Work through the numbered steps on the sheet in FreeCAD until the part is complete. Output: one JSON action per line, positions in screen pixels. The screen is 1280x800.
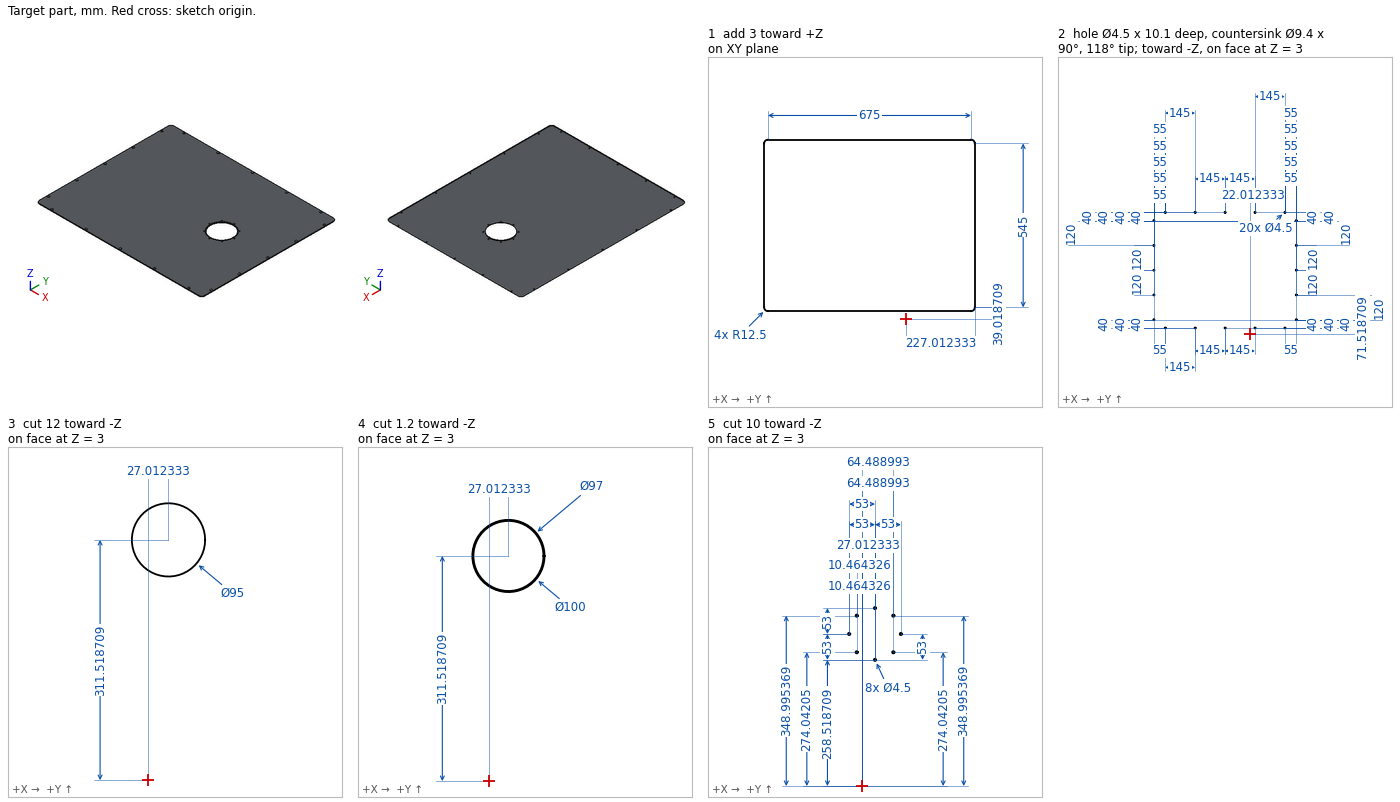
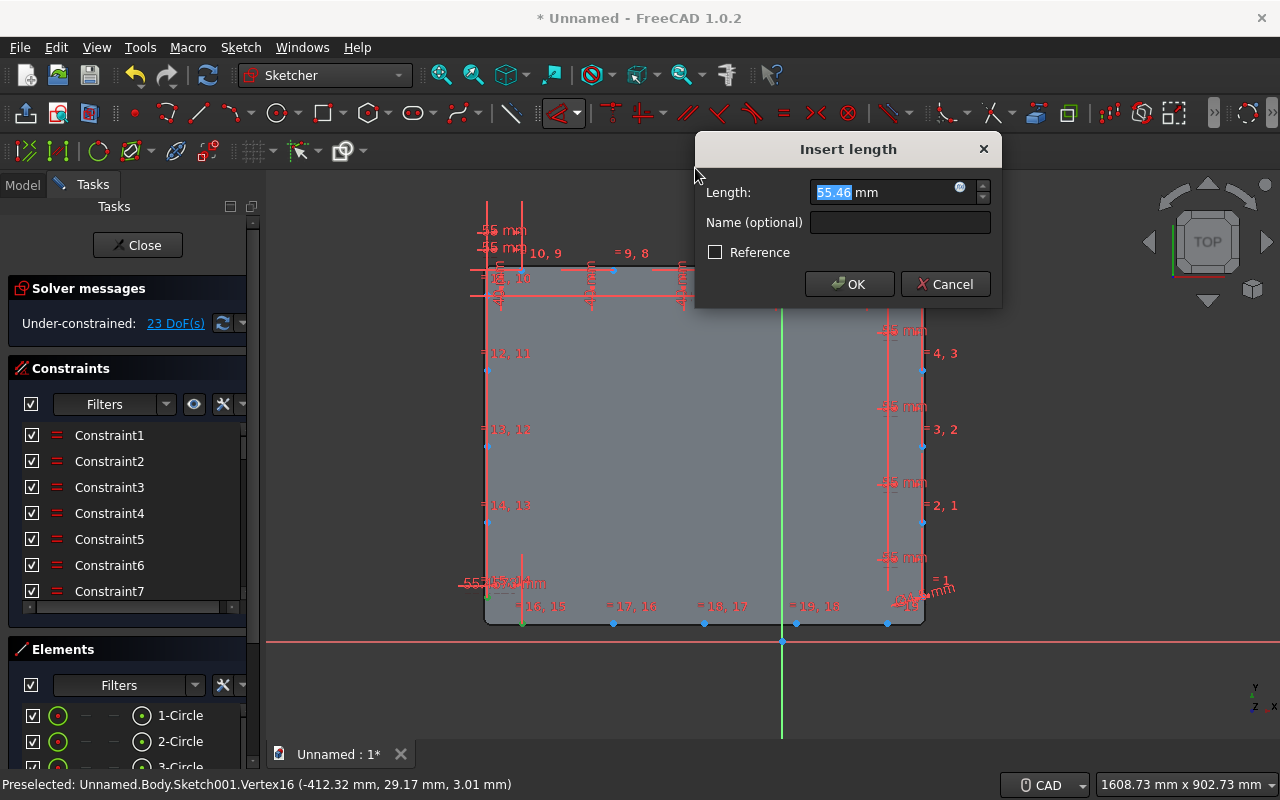
{"action": "type", "text": "55"}
{"action": "key", "text": "Return"}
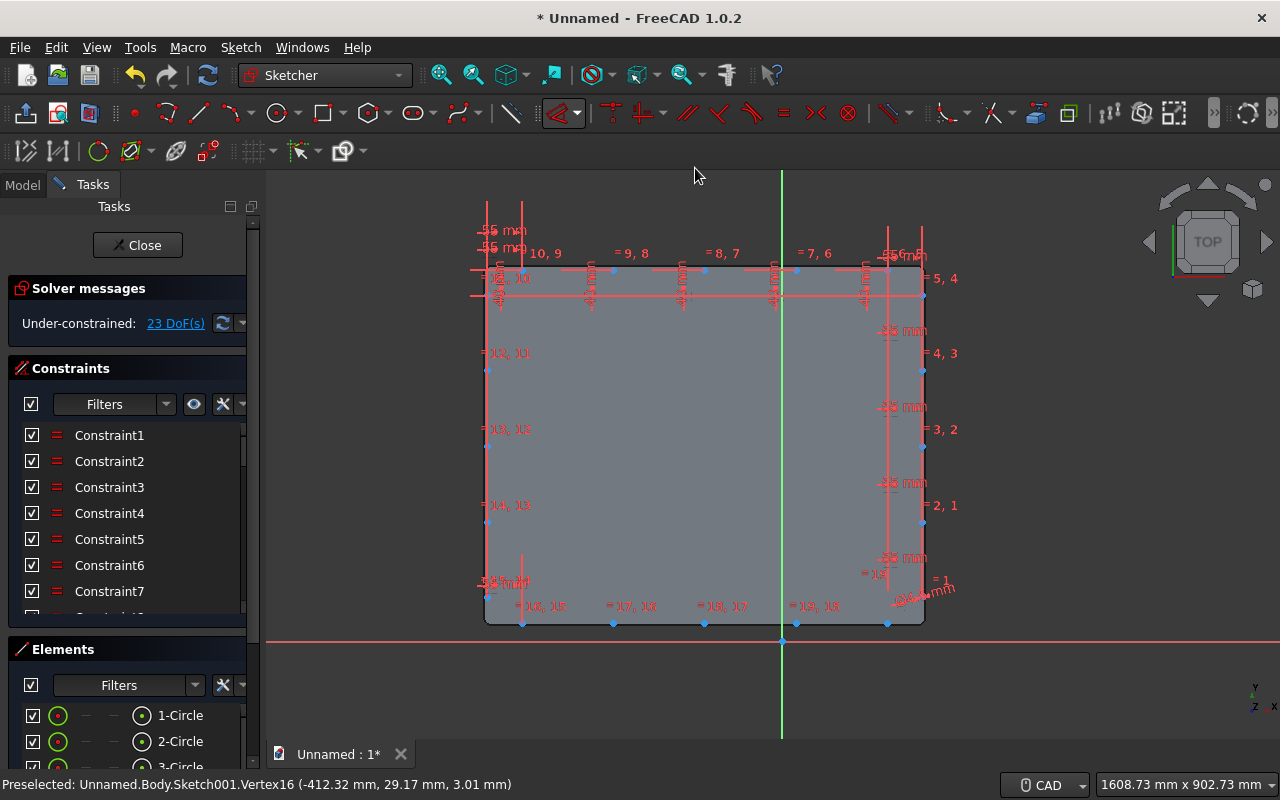
{"action": "scroll", "coordinate": [487, 597], "scroll_direction": "up", "scroll_amount": 3}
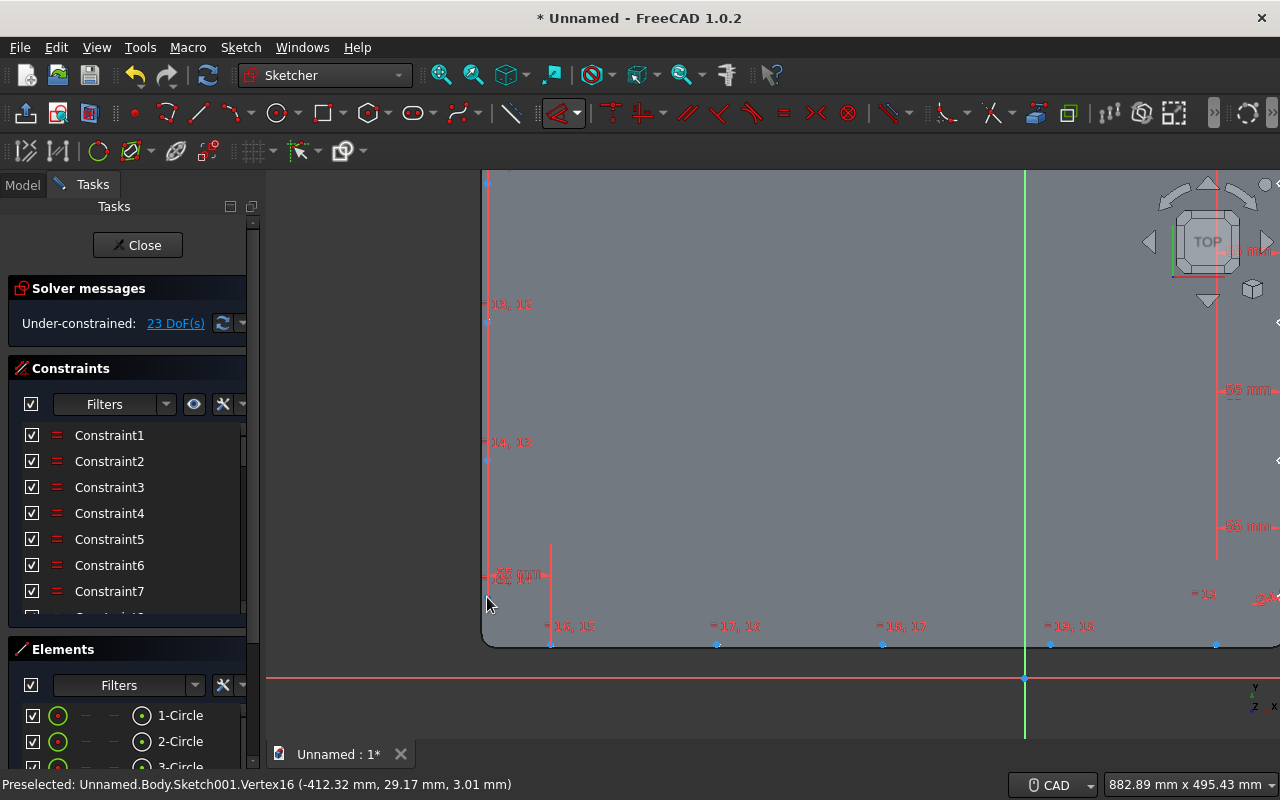
{"action": "left_click", "coordinate": [488, 597]}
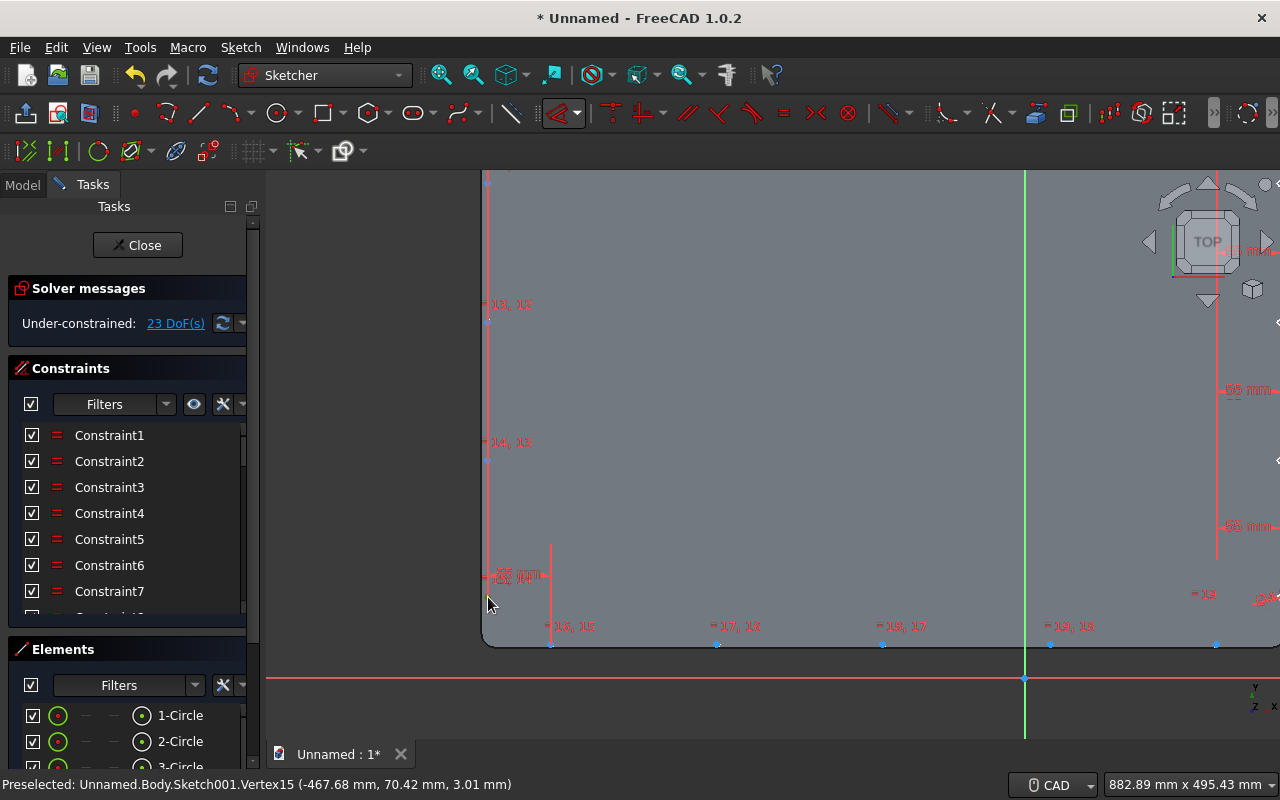
{"action": "left_click", "coordinate": [551, 645]}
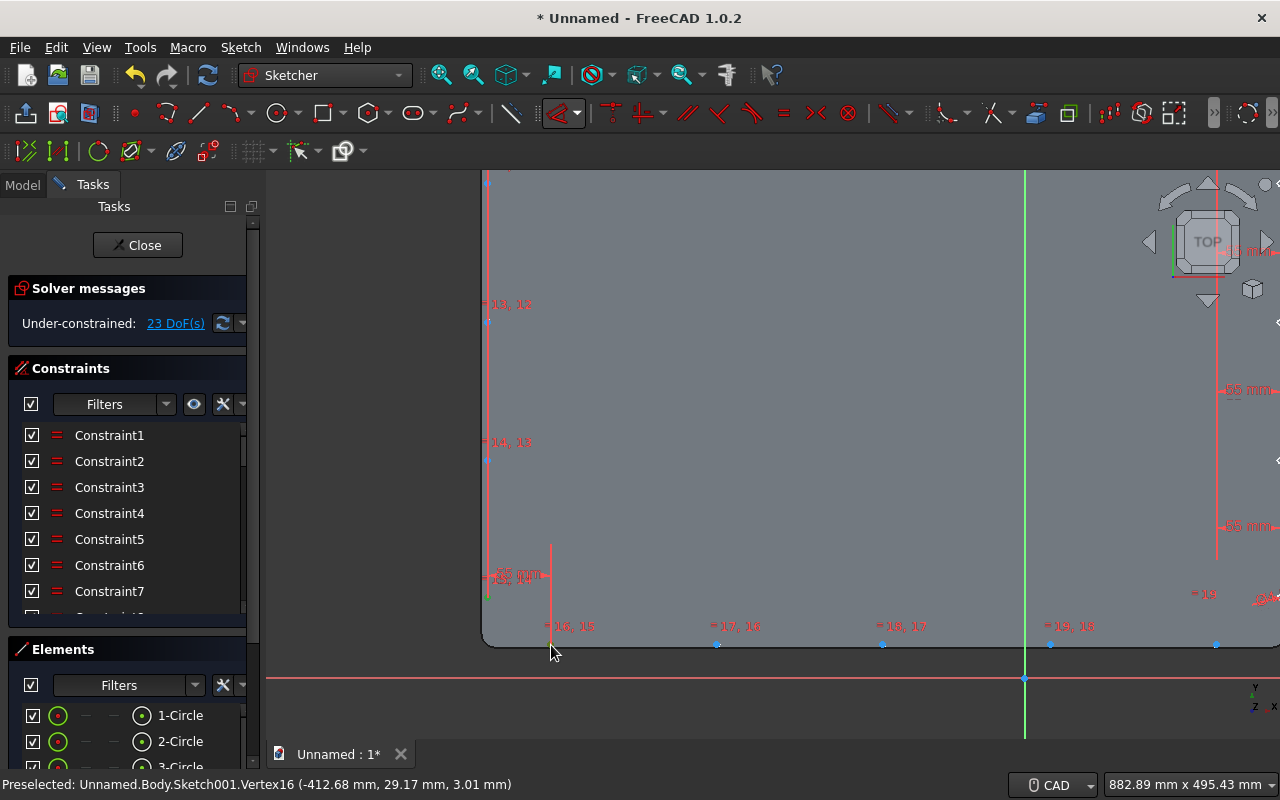
{"action": "key", "text": "i"}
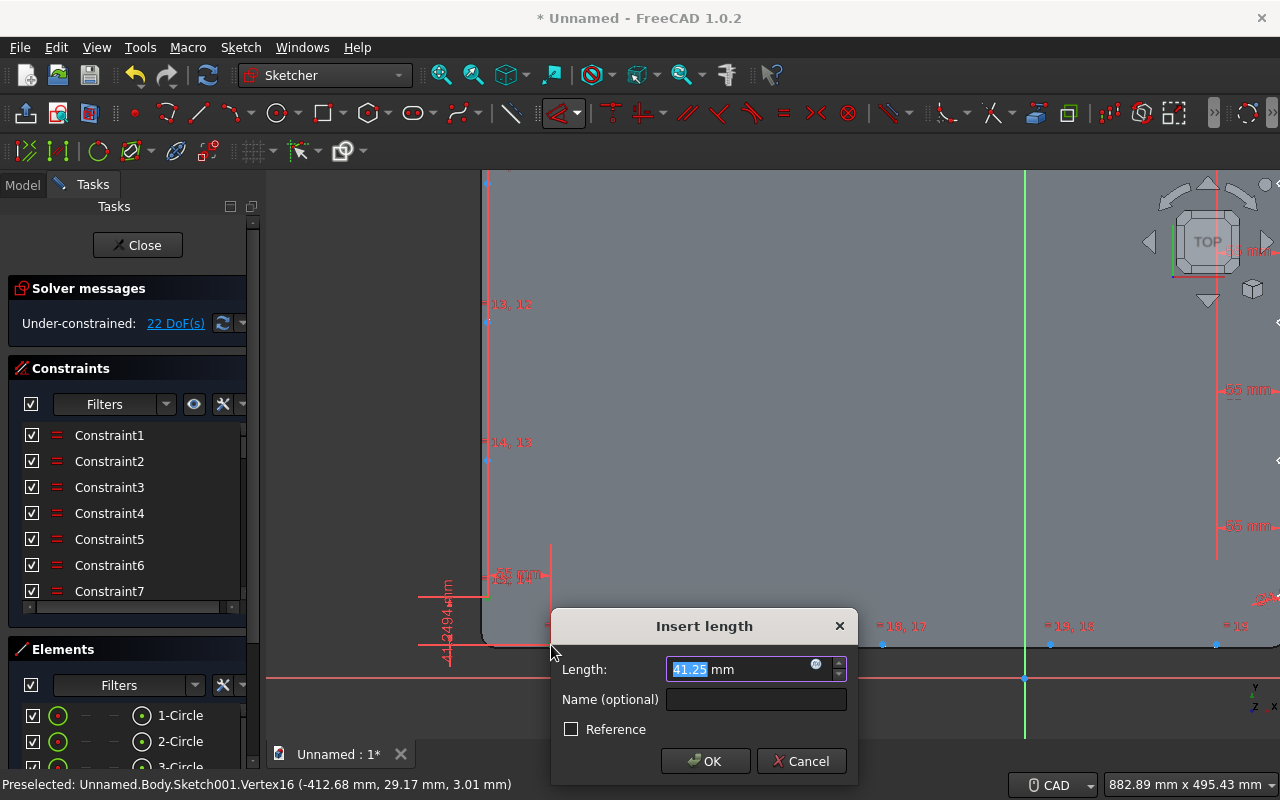
{"action": "type", "text": "40"}
{"action": "key", "text": "Return"}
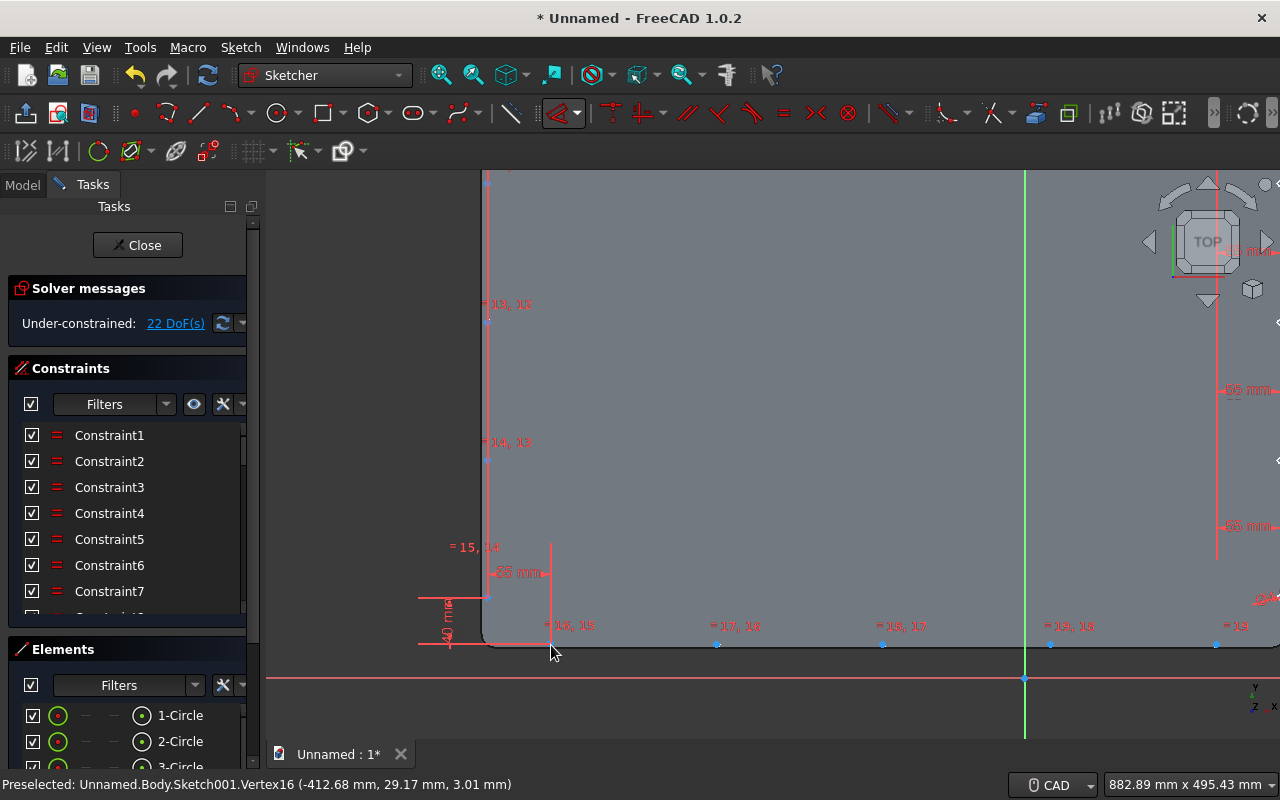
{"action": "left_click", "coordinate": [488, 598]}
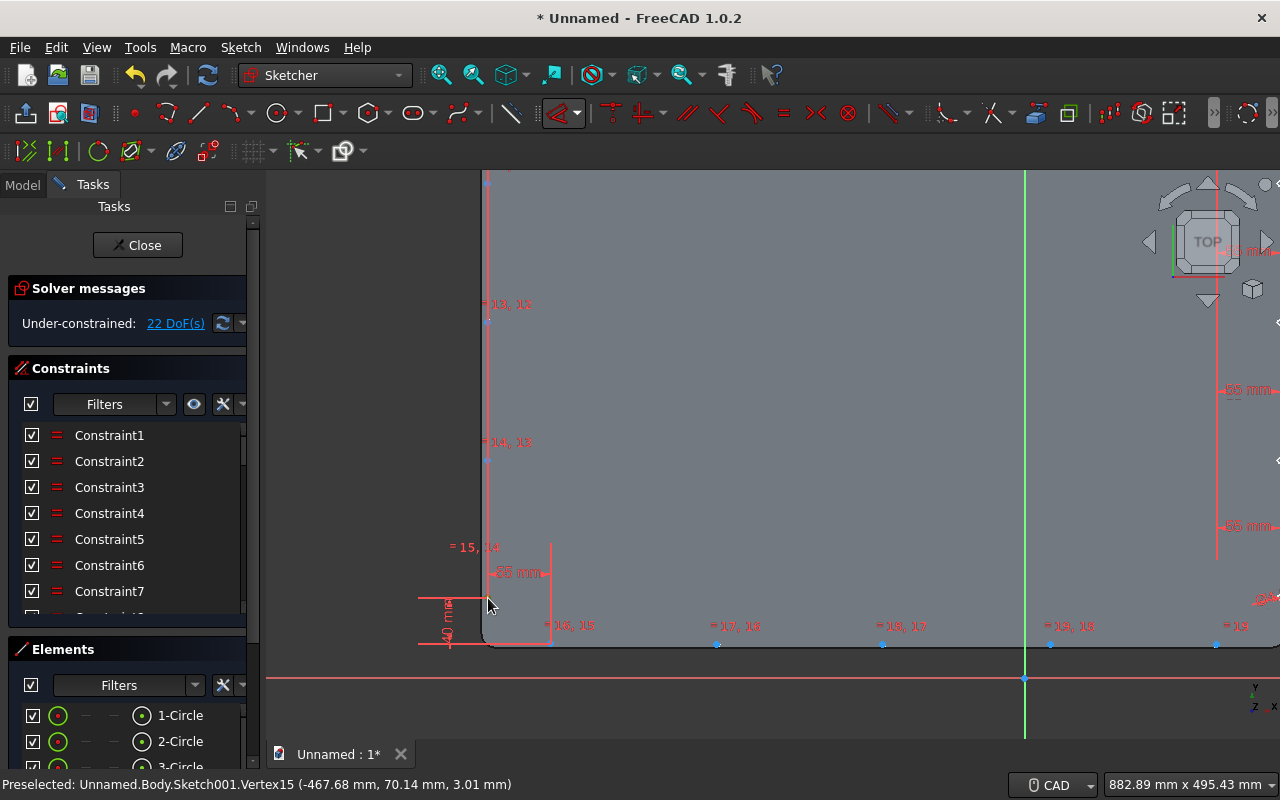
{"action": "left_click", "coordinate": [717, 645]}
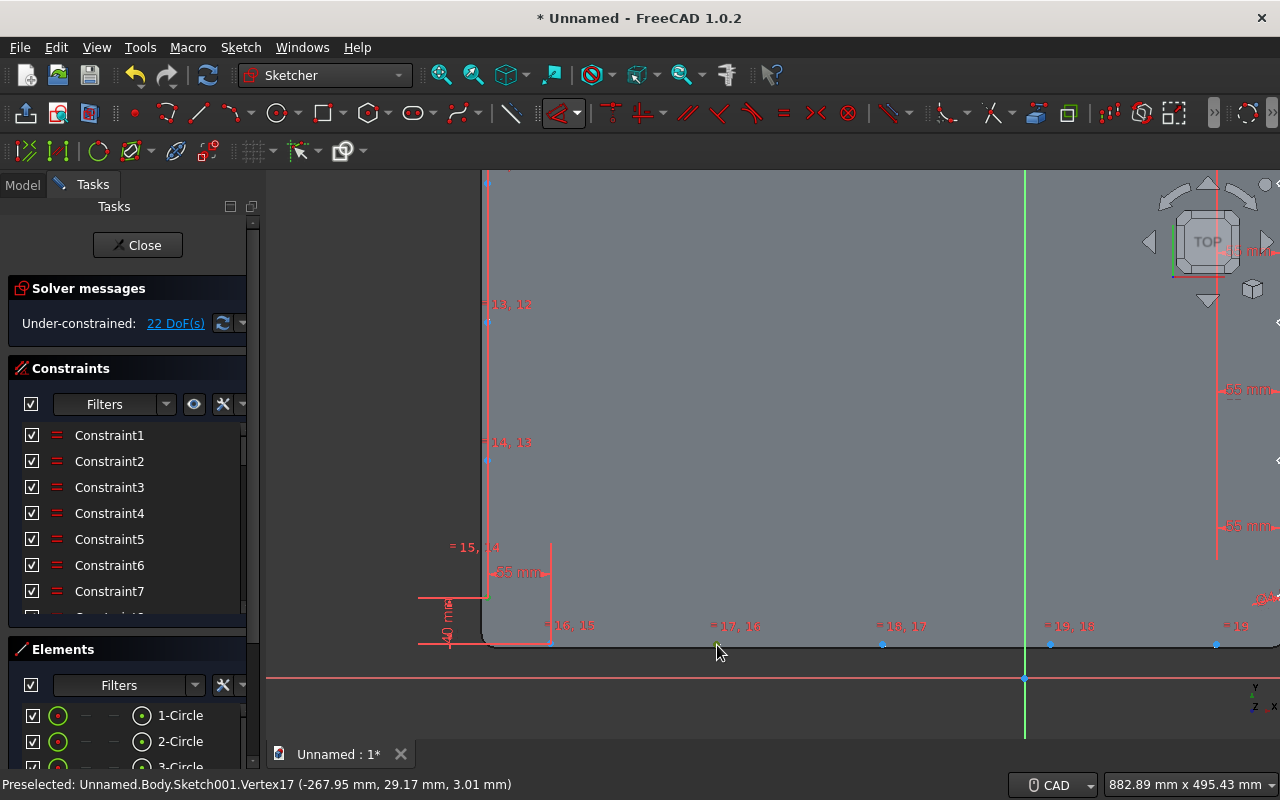
{"action": "left_click", "coordinate": [580, 114]}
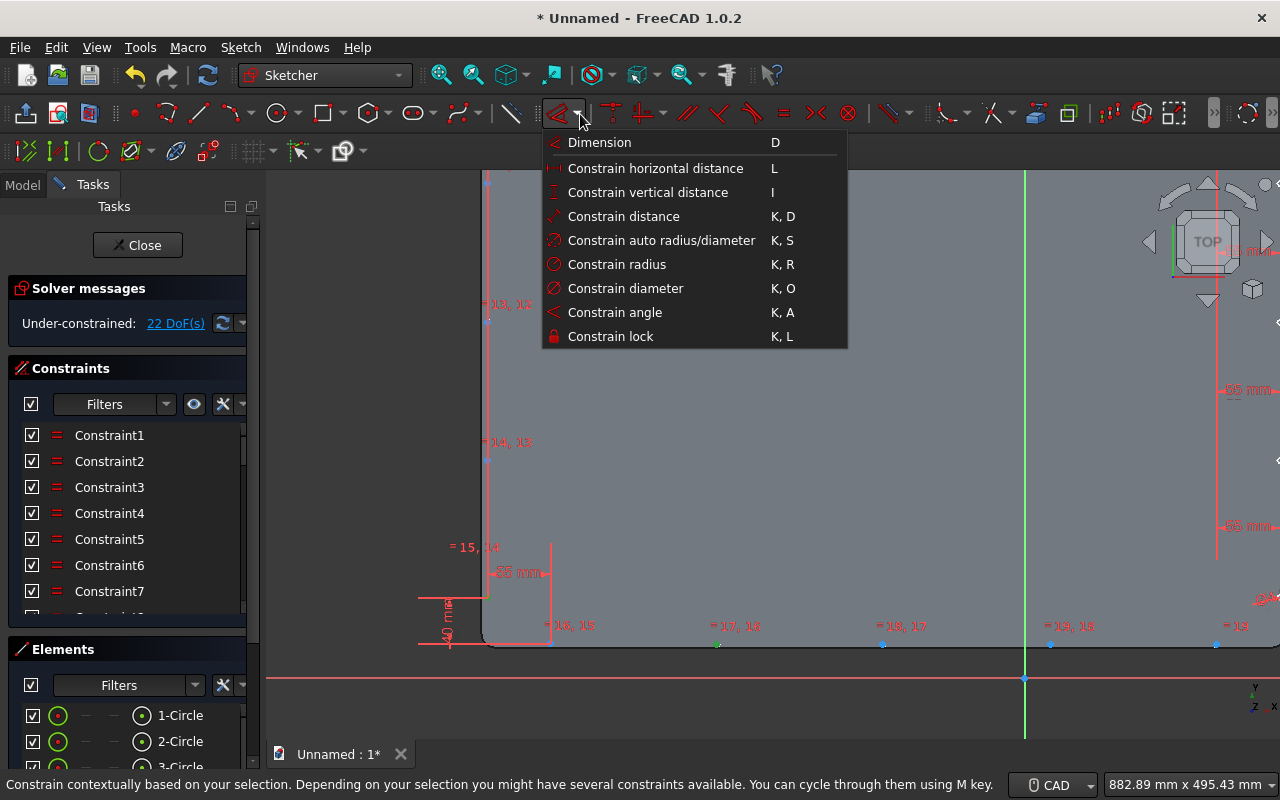
{"action": "left_click", "coordinate": [695, 192]}